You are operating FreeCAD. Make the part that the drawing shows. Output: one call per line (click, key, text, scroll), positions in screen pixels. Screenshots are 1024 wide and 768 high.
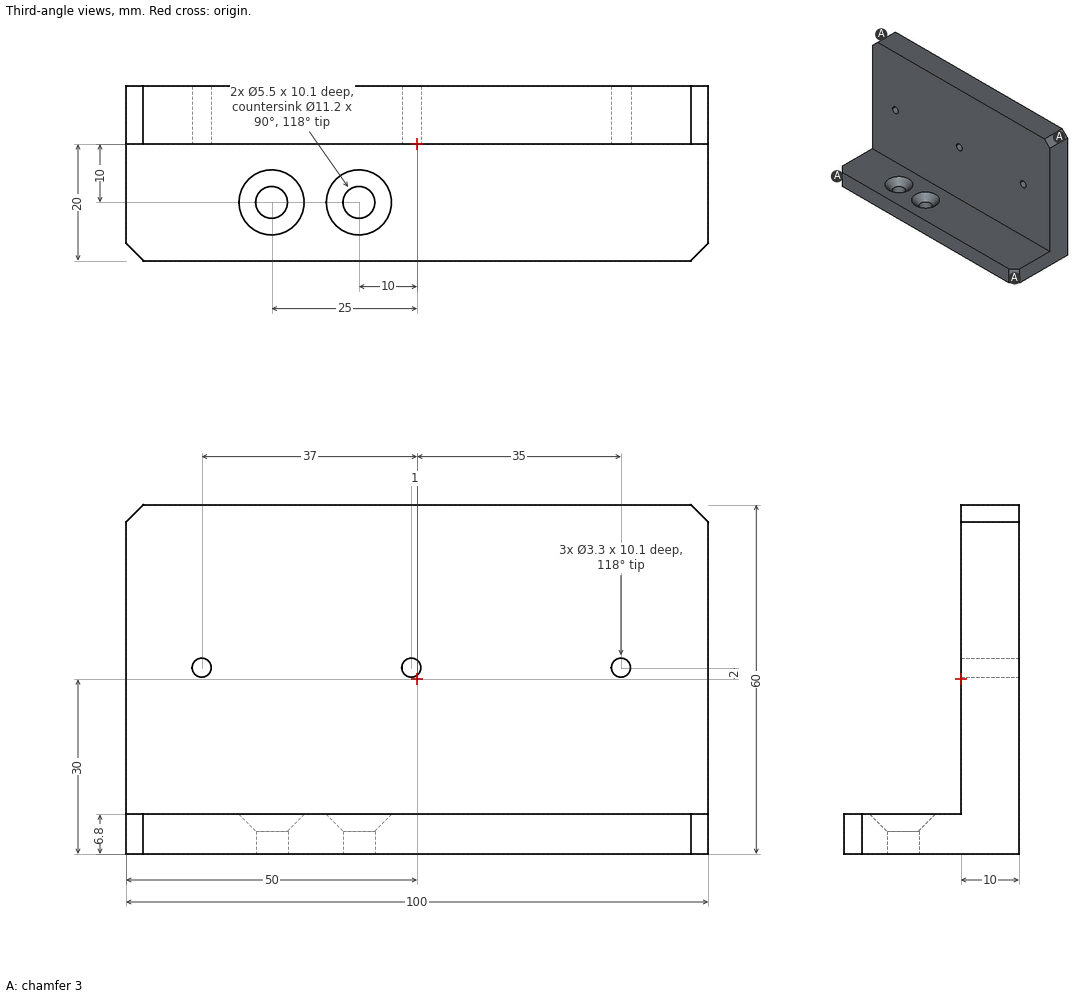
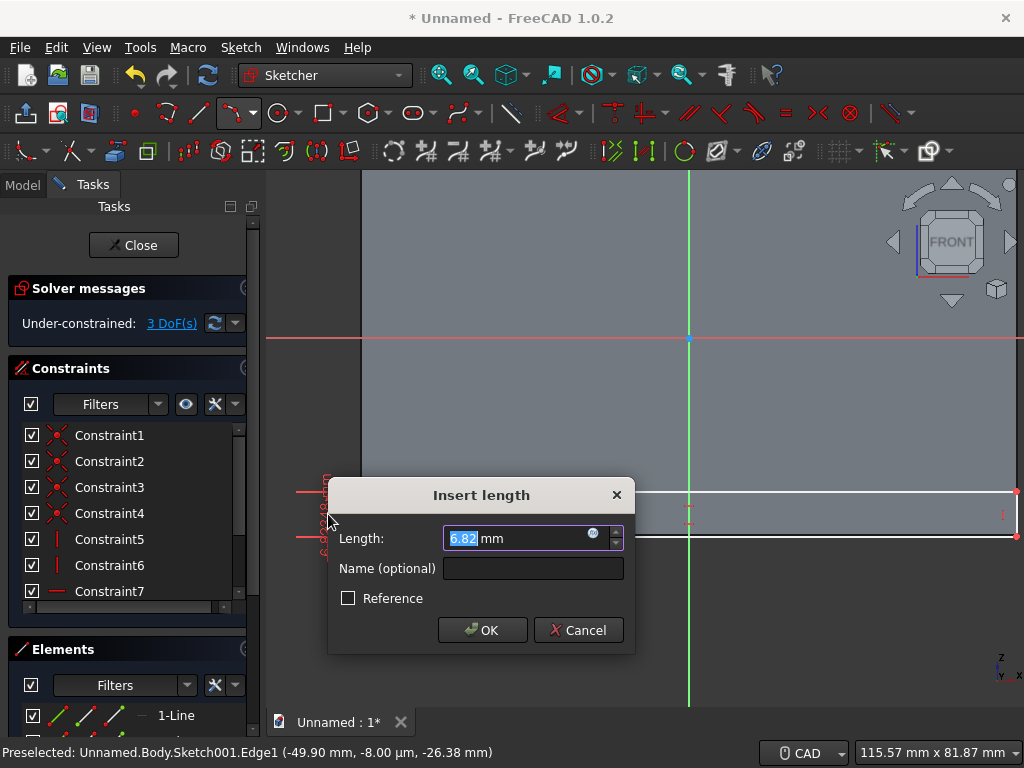
text(6.8)
key(Return)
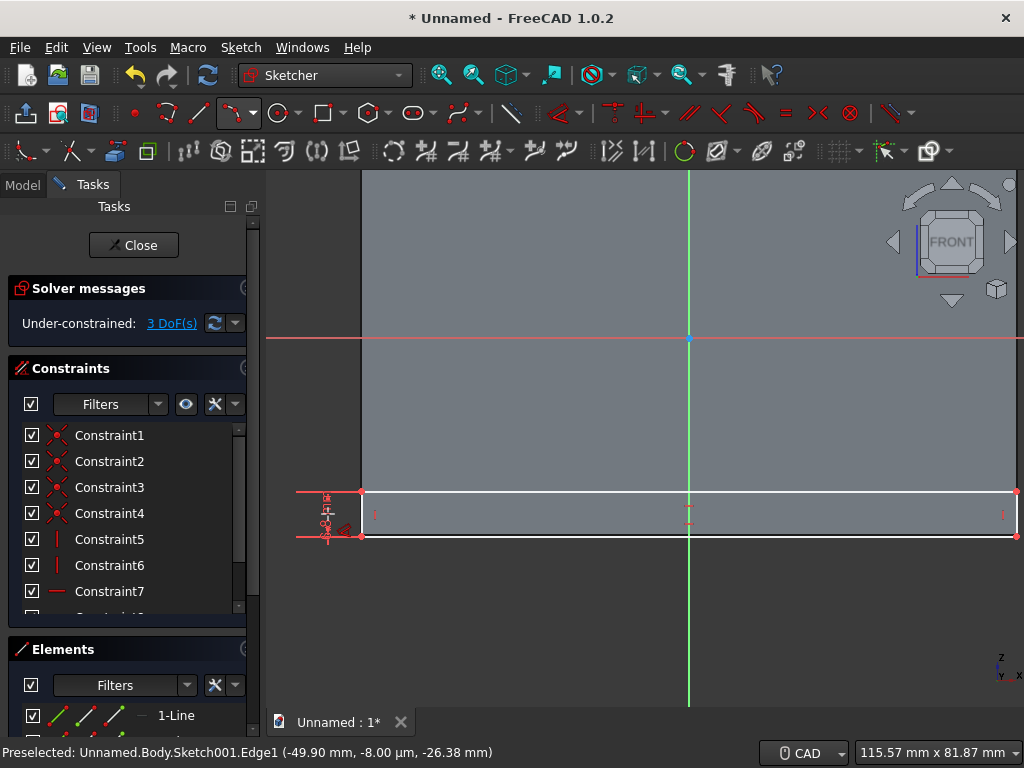
click(558, 537)
click(610, 571)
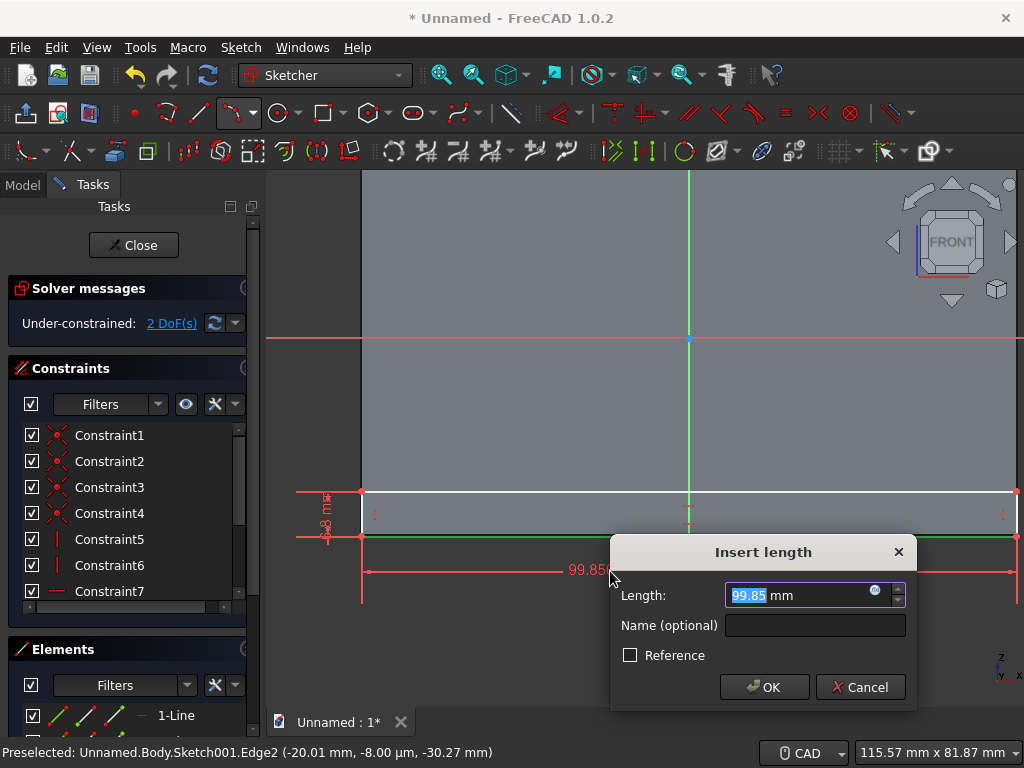
text(100)
key(Return)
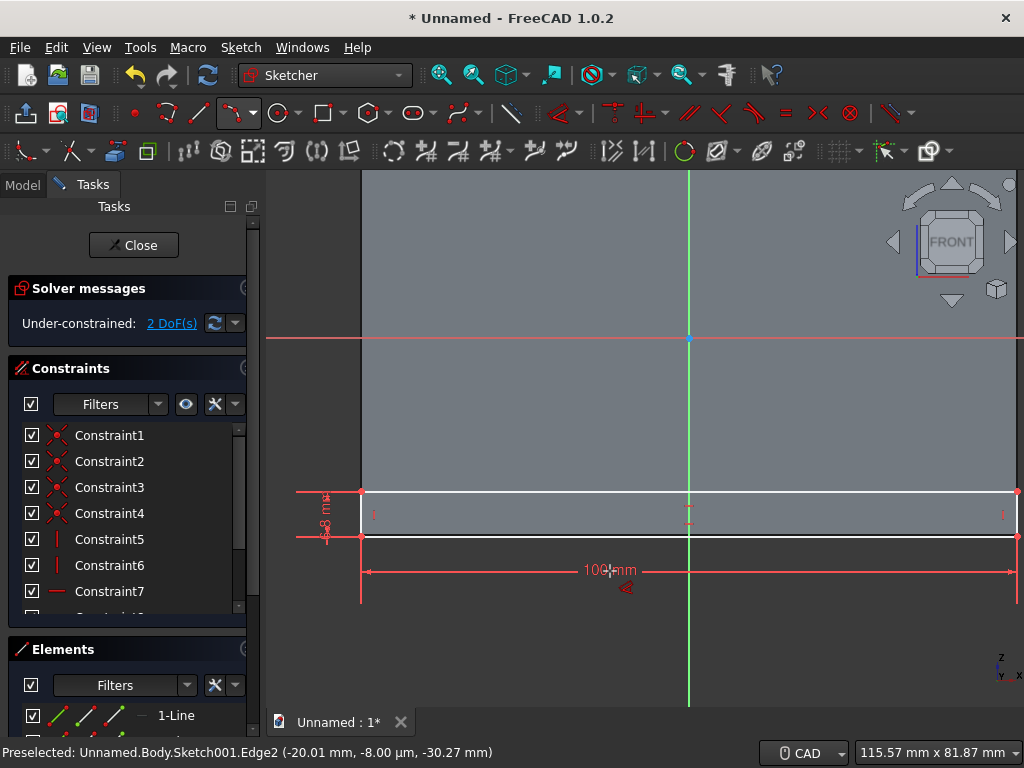
click(361, 492)
click(525, 304)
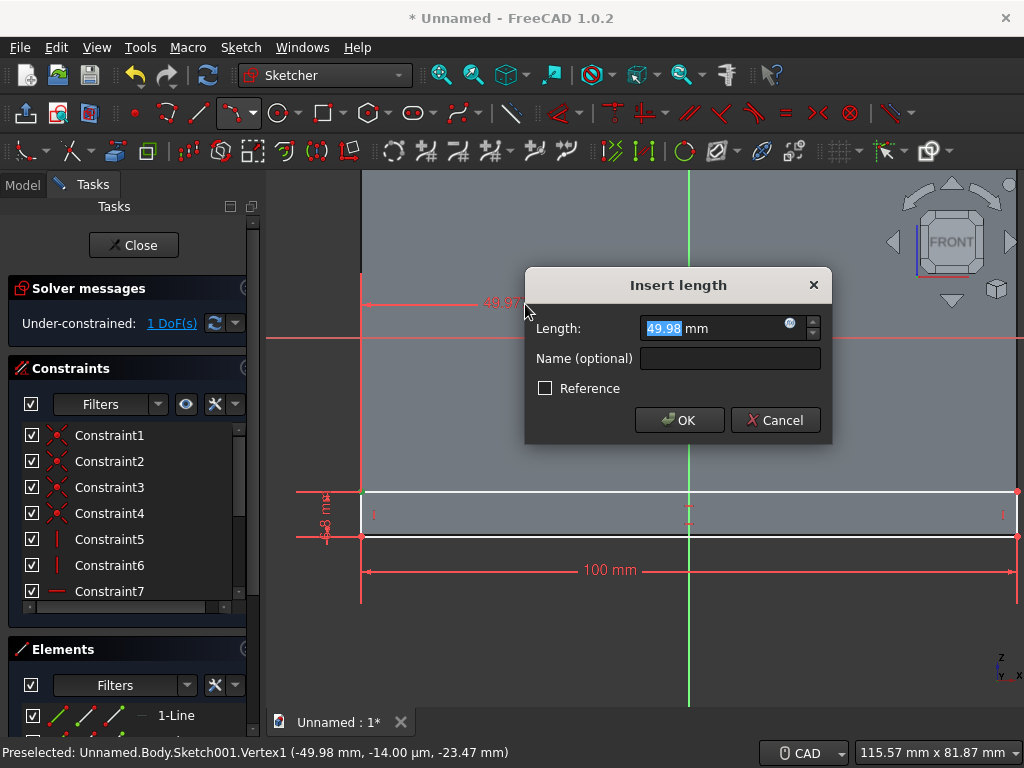
text(50)
key(Return)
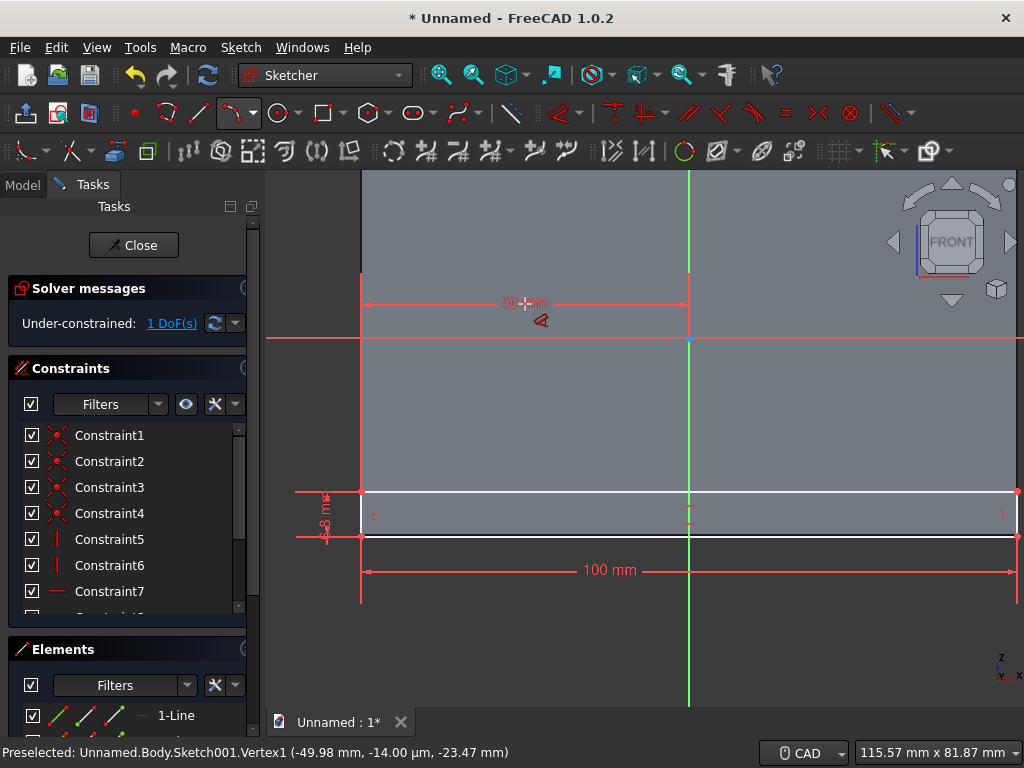
click(361, 537)
click(327, 437)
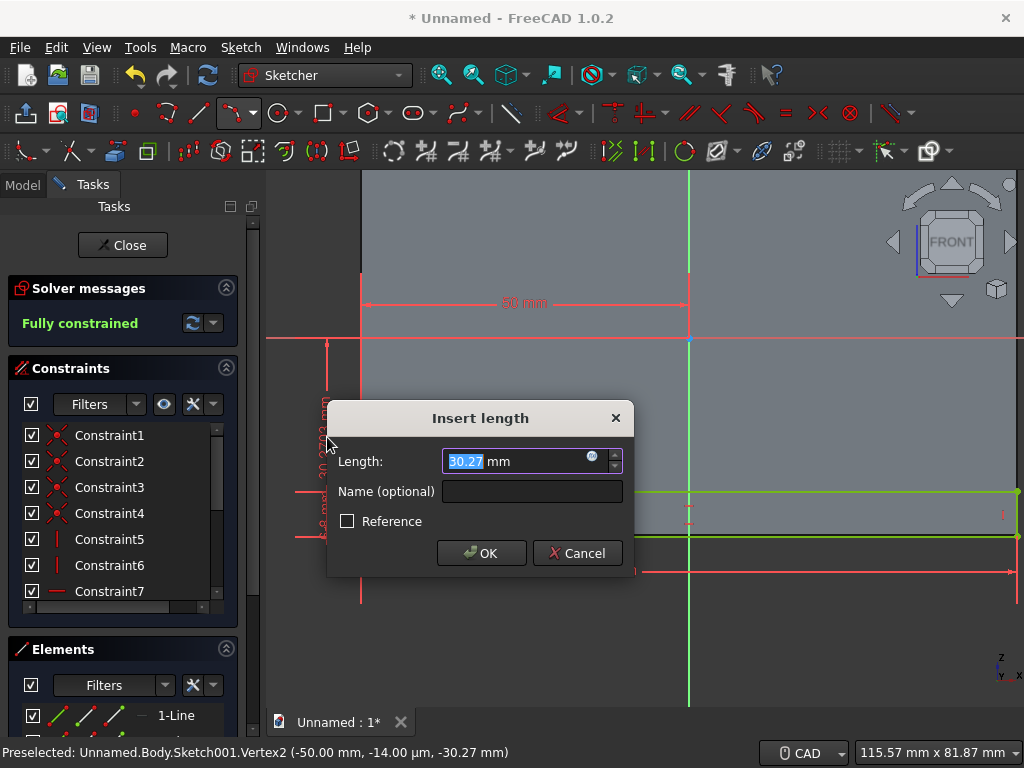
text(30)
key(Return)
key(Escape)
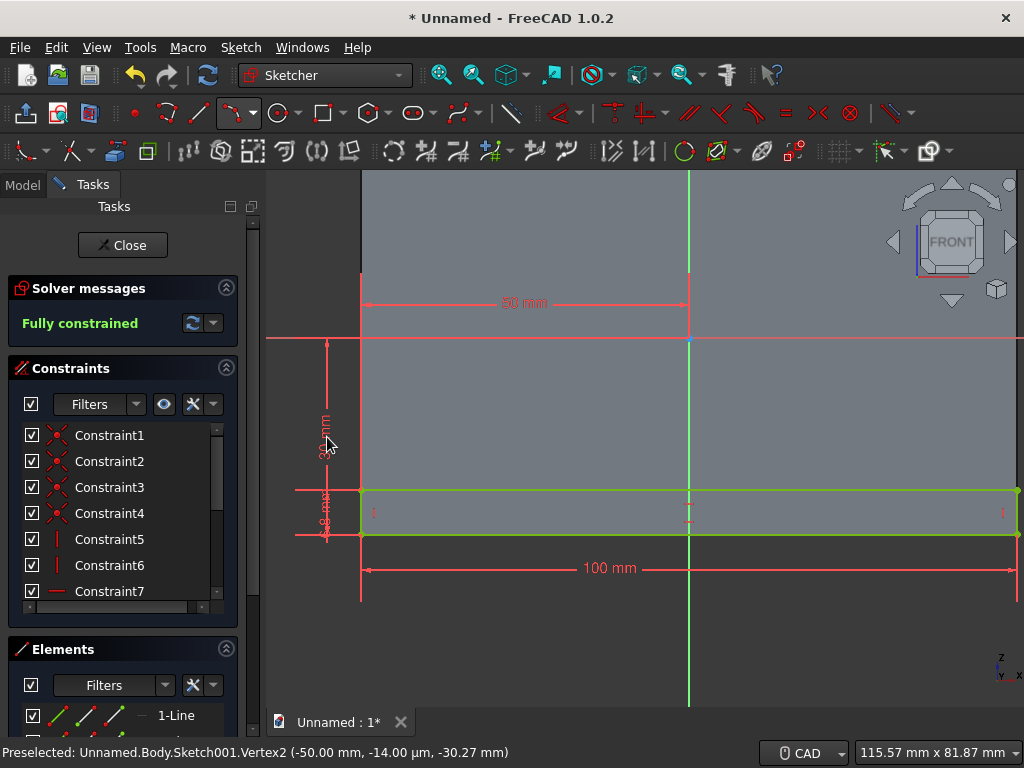
click(123, 245)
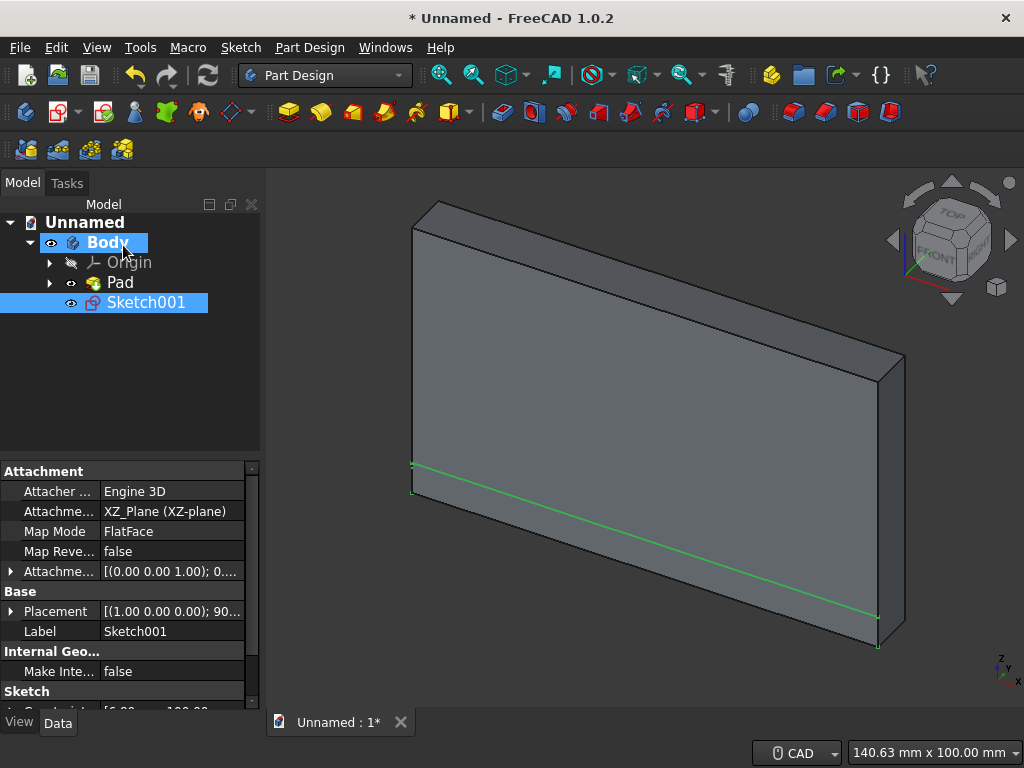
click(290, 112)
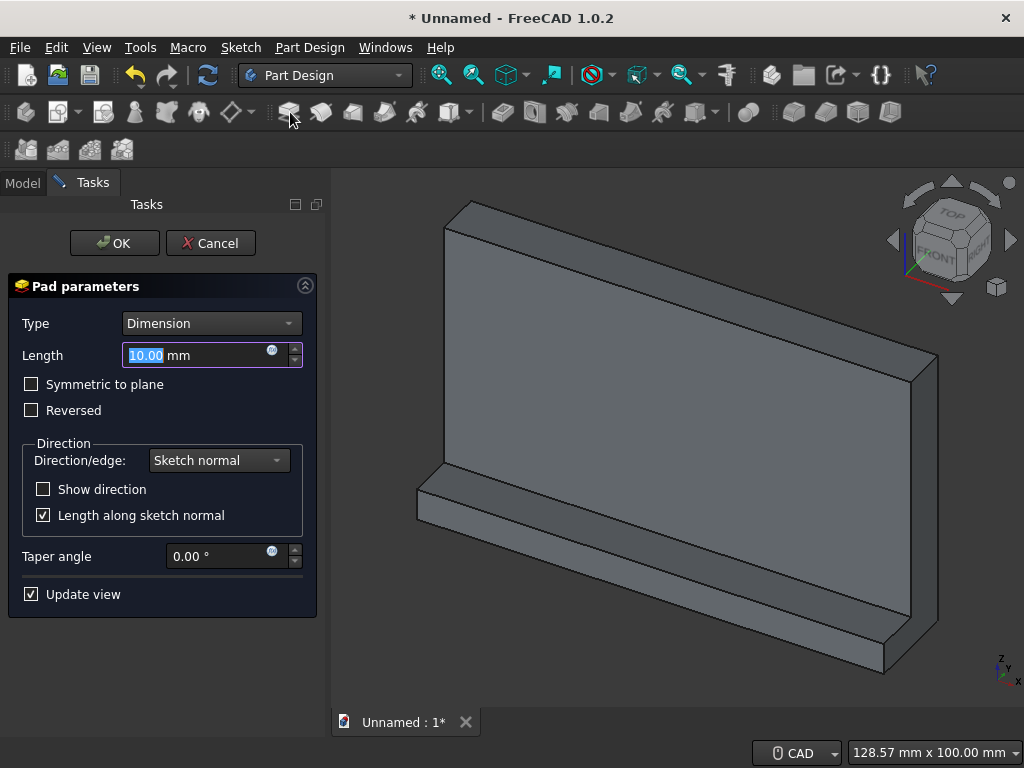
text(20)
key(Tab)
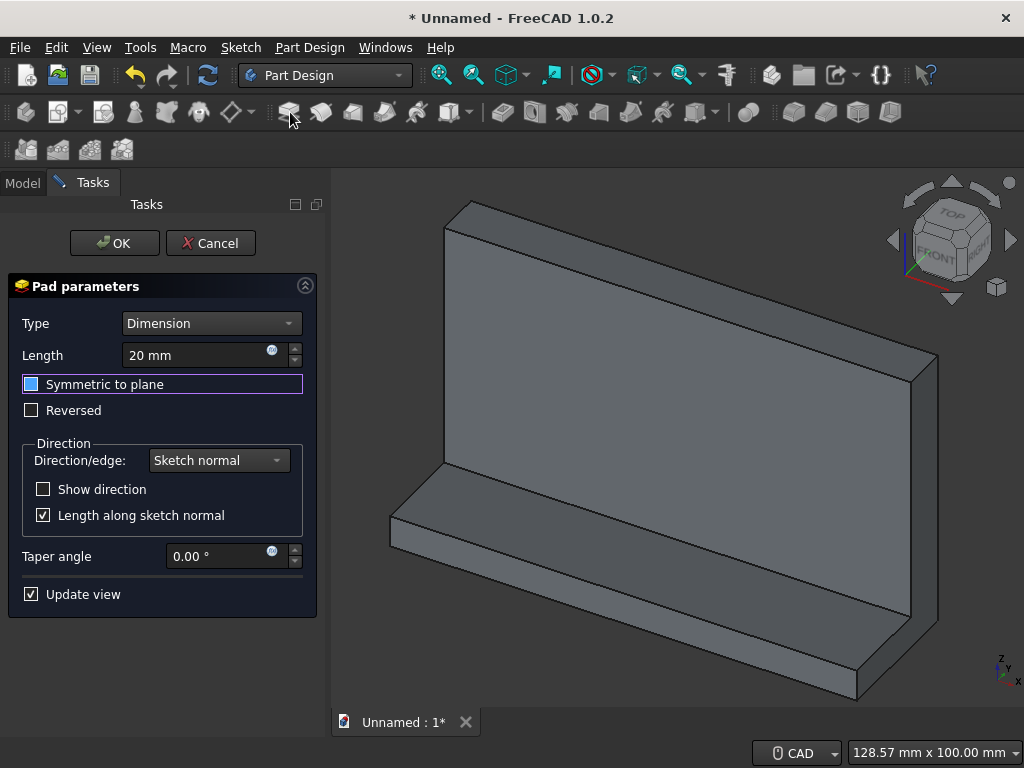
click(115, 243)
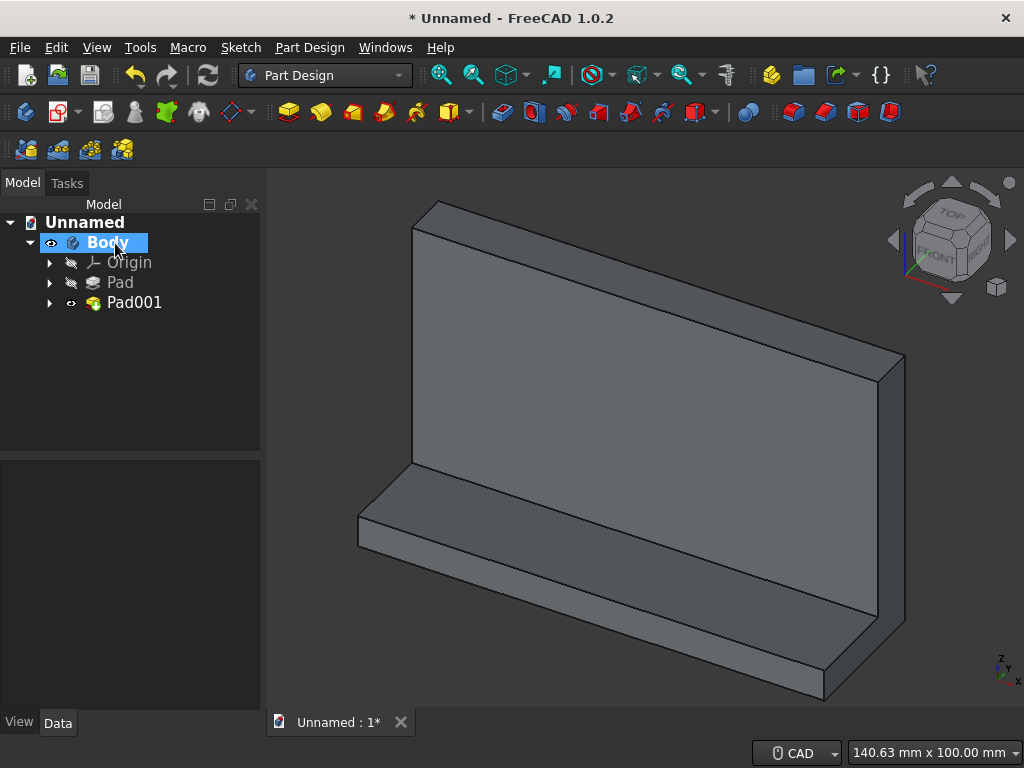
click(824, 676)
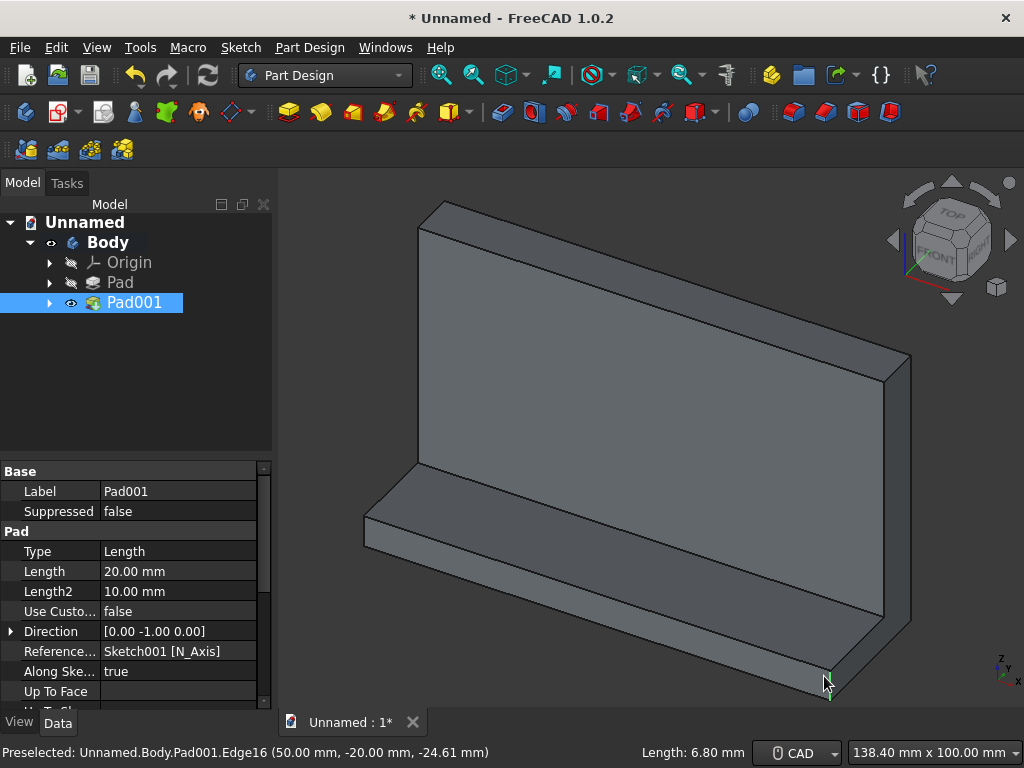
click(898, 368, ctrl)